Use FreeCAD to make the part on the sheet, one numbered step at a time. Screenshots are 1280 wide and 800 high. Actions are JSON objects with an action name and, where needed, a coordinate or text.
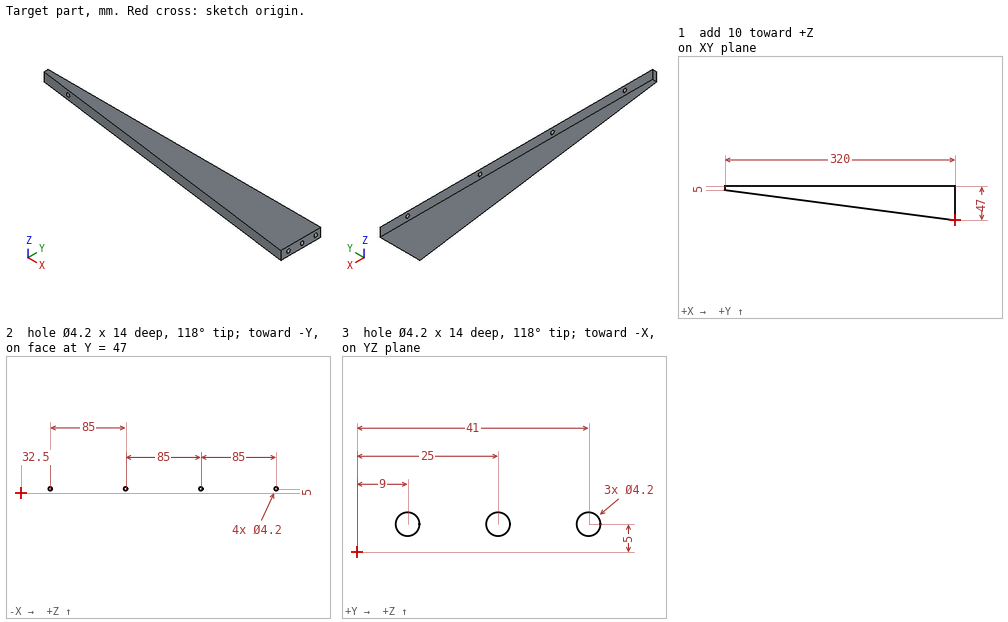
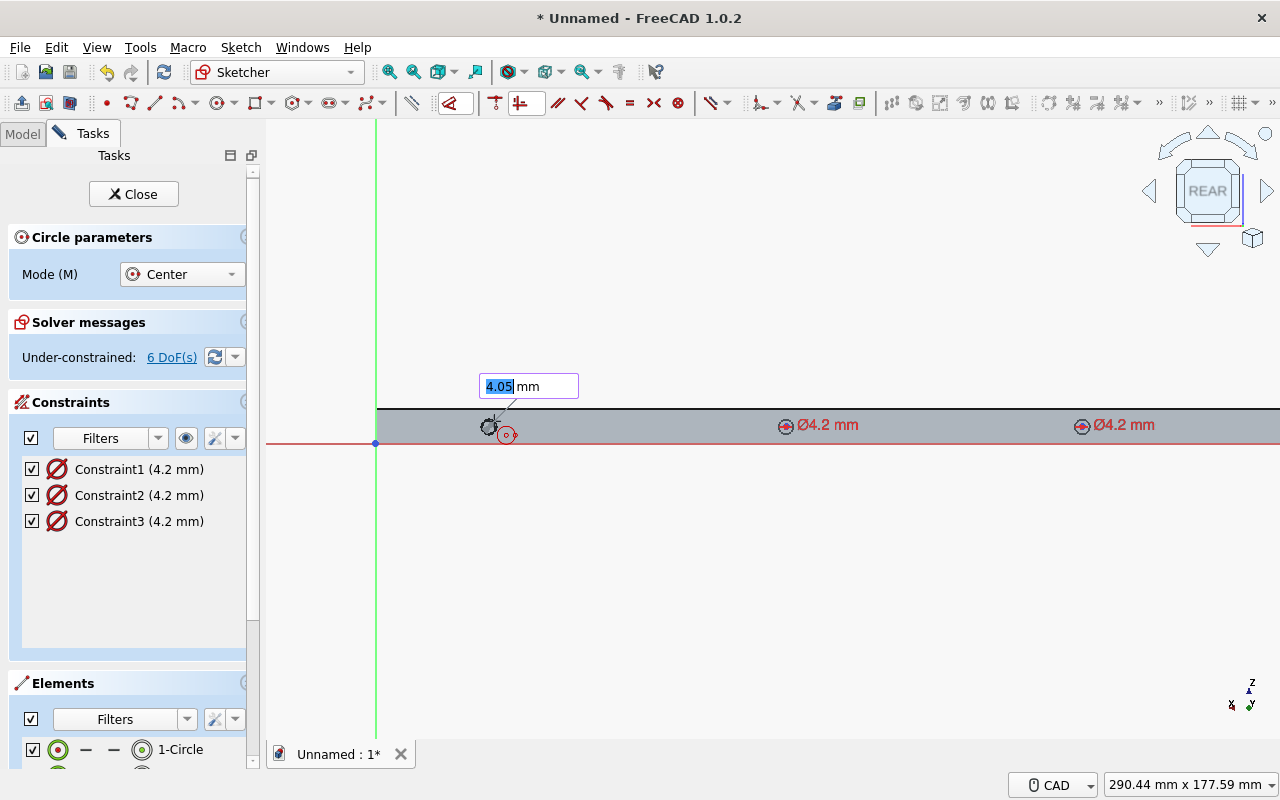
{"action": "type", "text": "4.2"}
{"action": "key", "text": "Return"}
{"action": "key", "text": "Escape"}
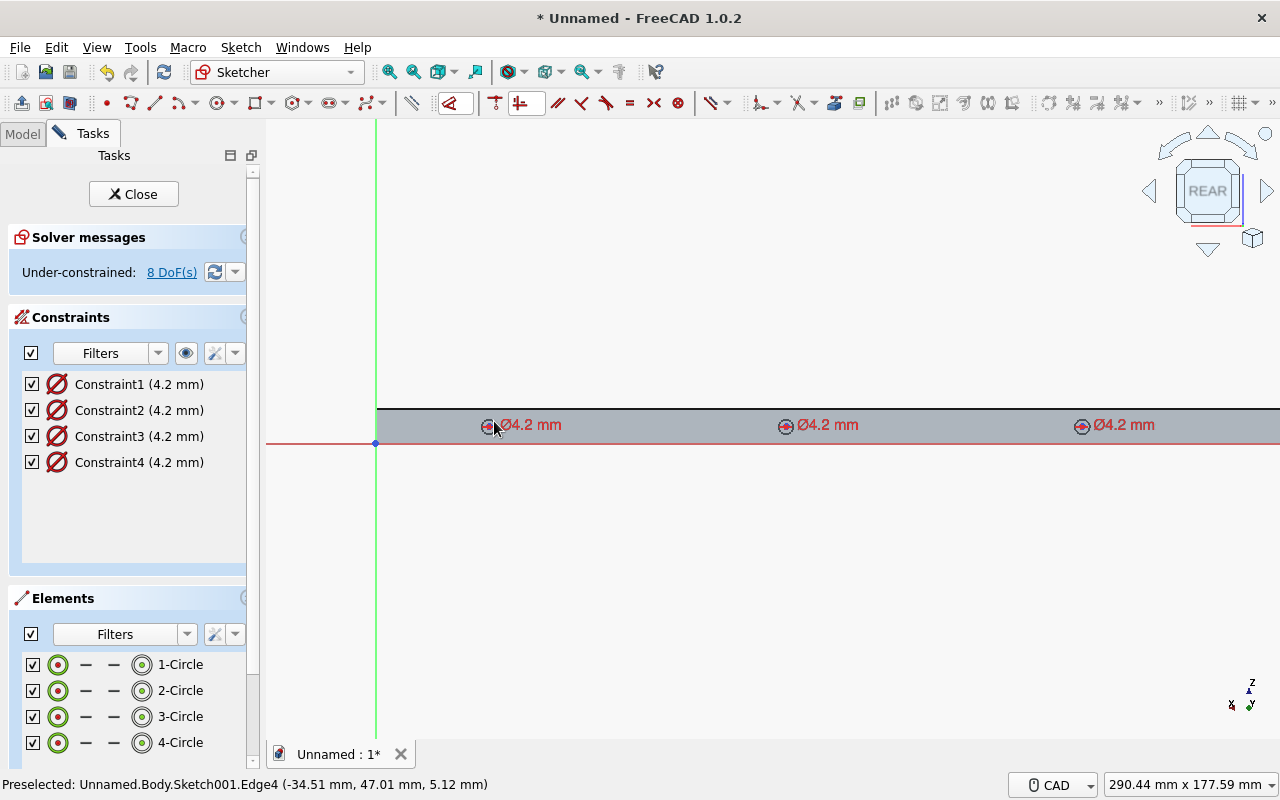
{"action": "scroll", "coordinate": [489, 426], "scroll_direction": "down", "scroll_amount": 3}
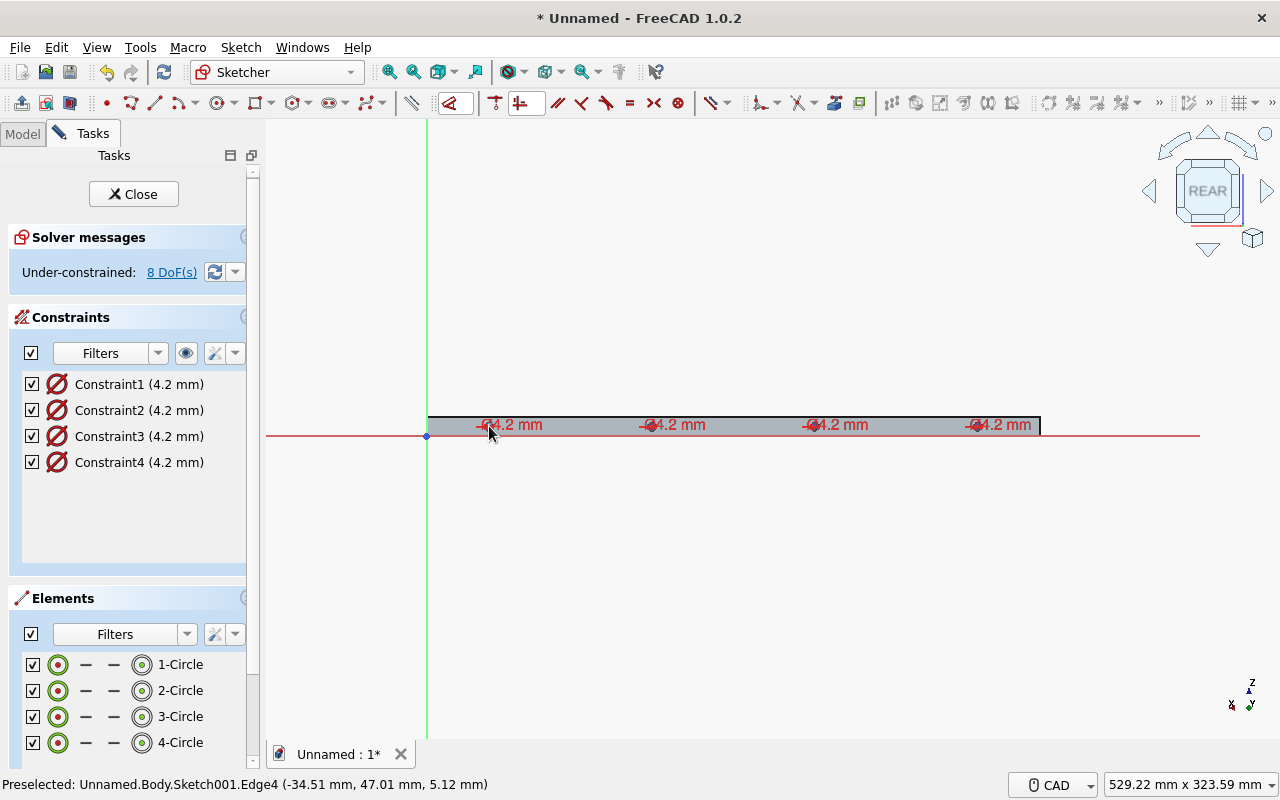
{"action": "left_click", "coordinate": [978, 427]}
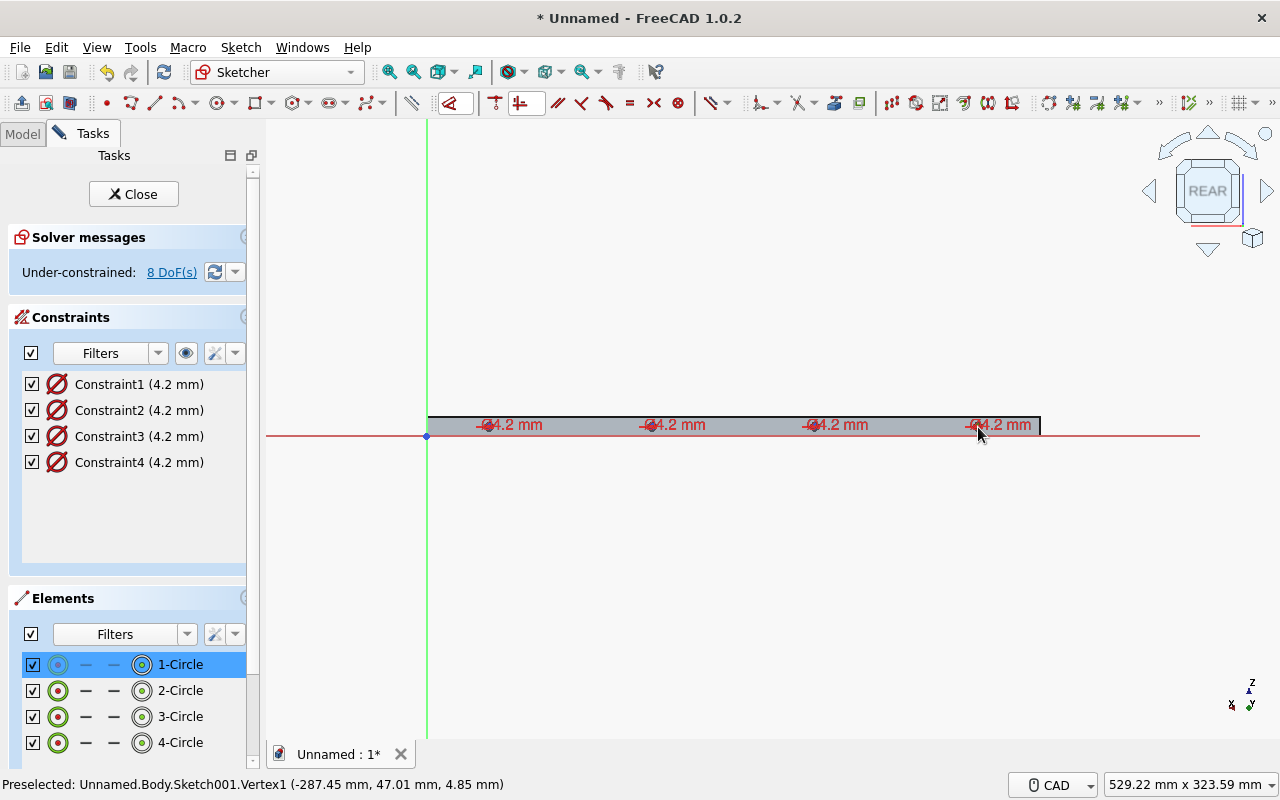
{"action": "left_click", "coordinate": [815, 427]}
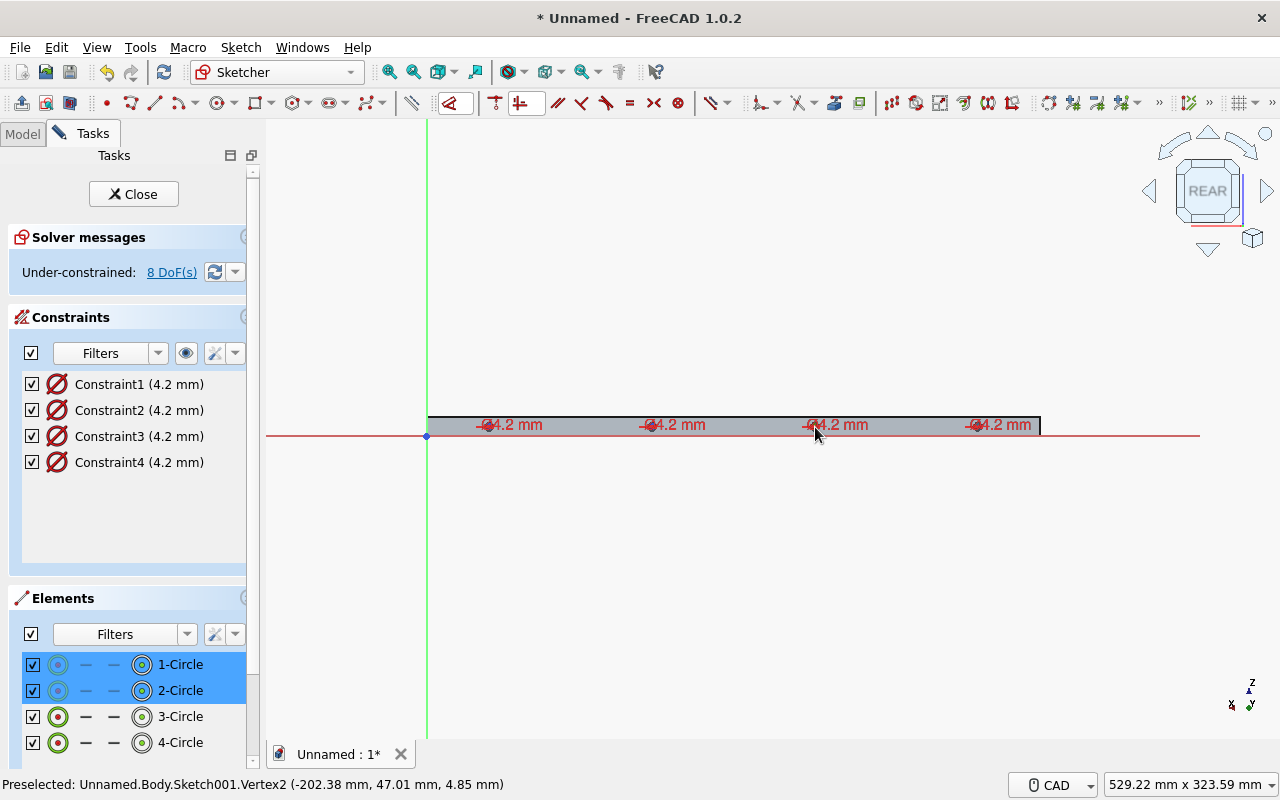
{"action": "key", "text": "h"}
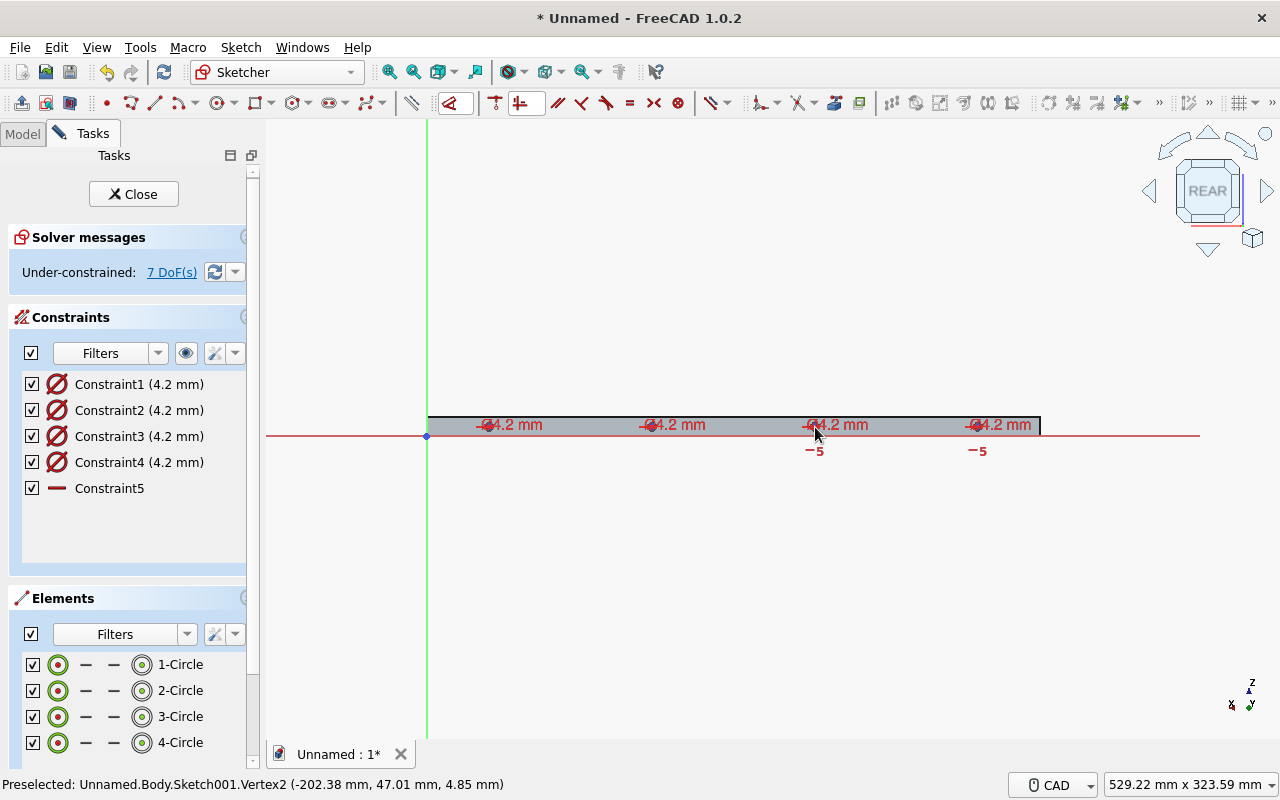
{"action": "left_click", "coordinate": [815, 427]}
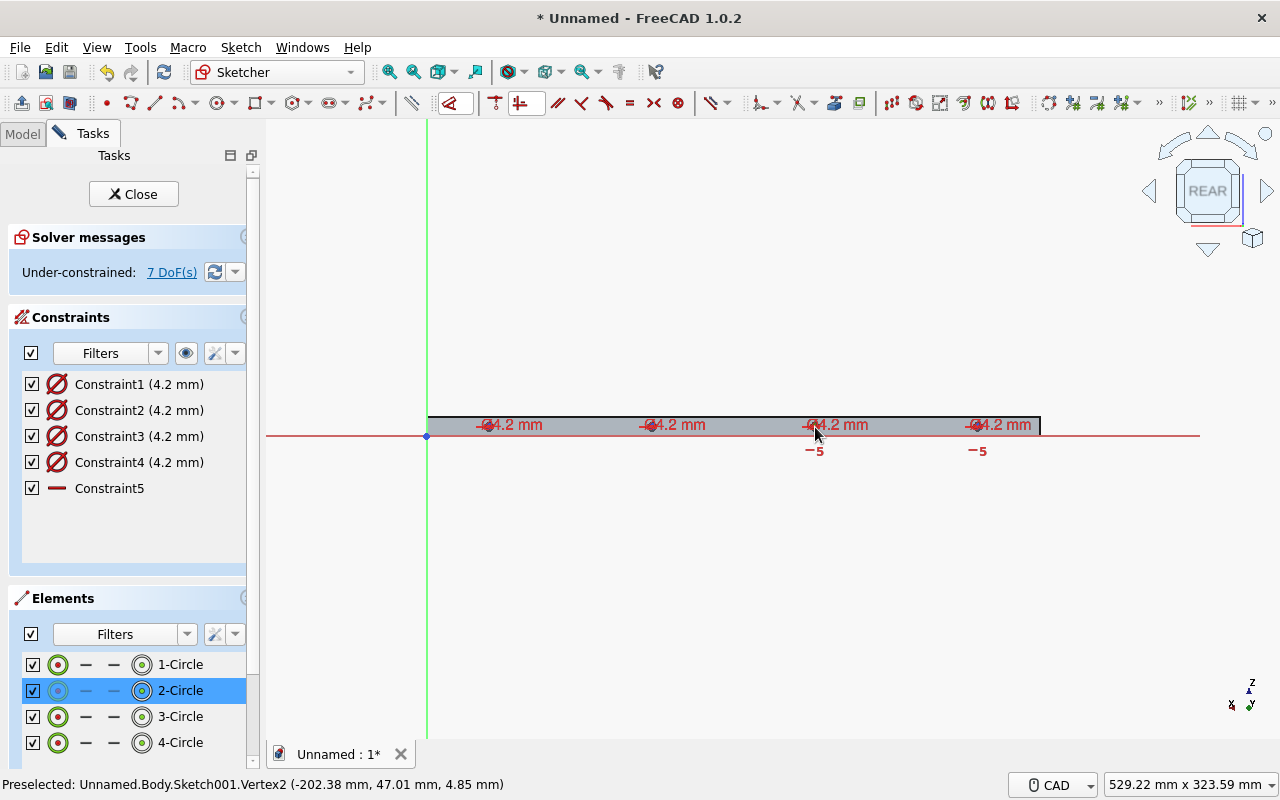
{"action": "left_click", "coordinate": [652, 427]}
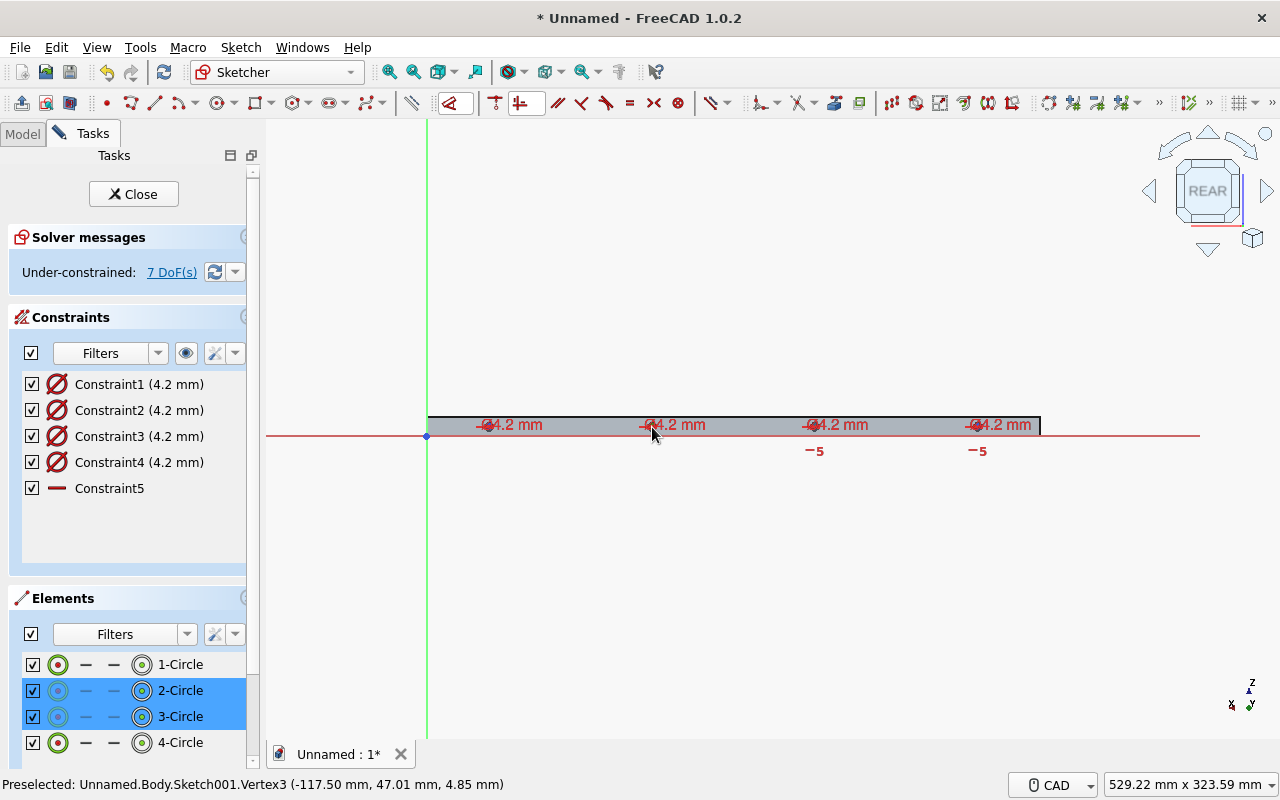
{"action": "left_click", "coordinate": [540, 104]}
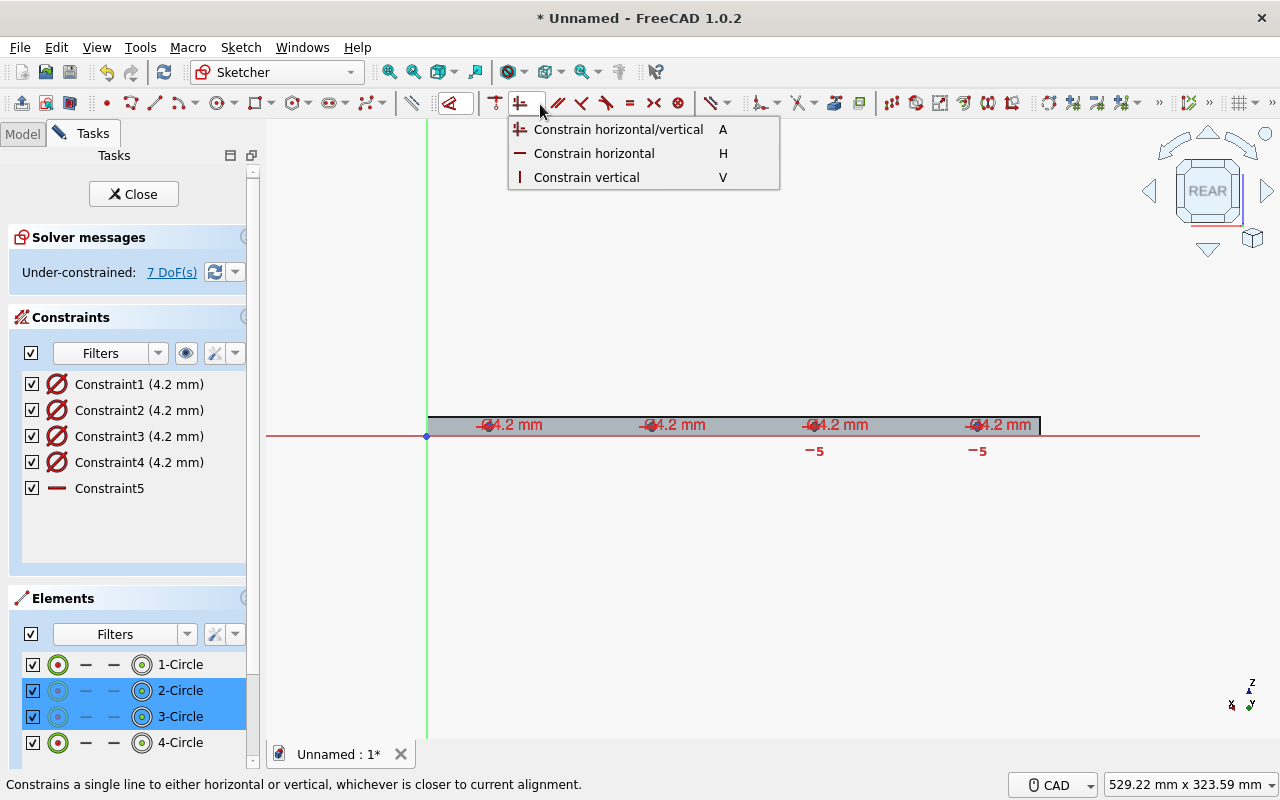
{"action": "left_click", "coordinate": [644, 153]}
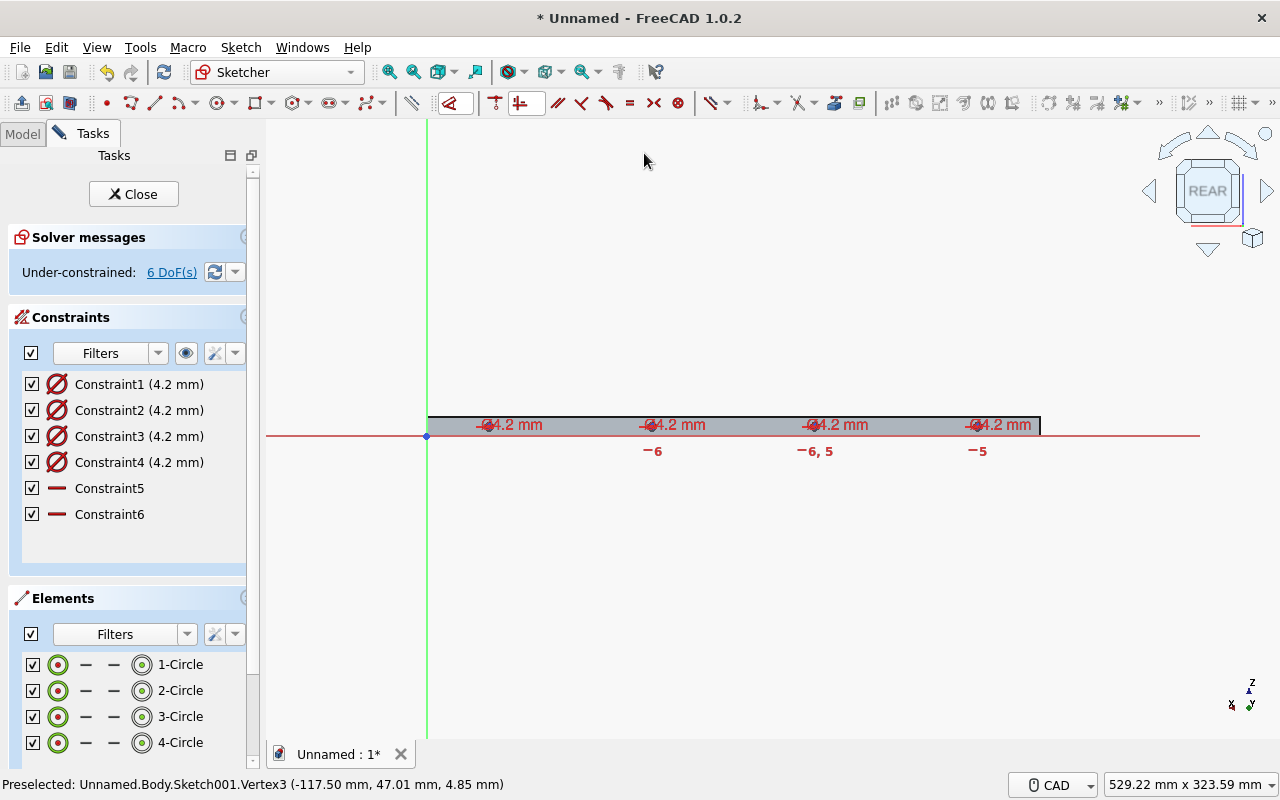
{"action": "left_click", "coordinate": [652, 427]}